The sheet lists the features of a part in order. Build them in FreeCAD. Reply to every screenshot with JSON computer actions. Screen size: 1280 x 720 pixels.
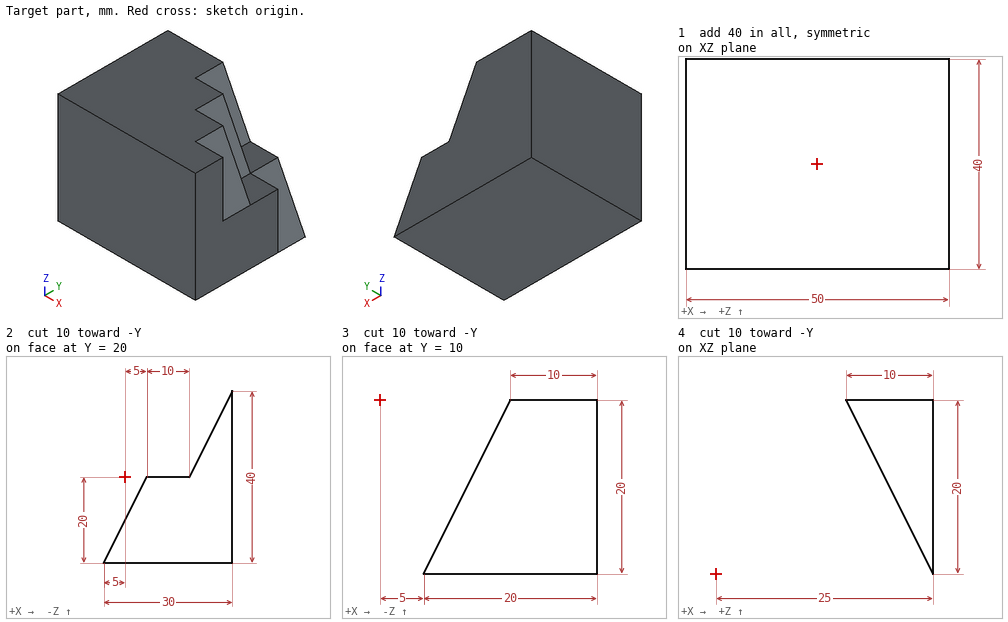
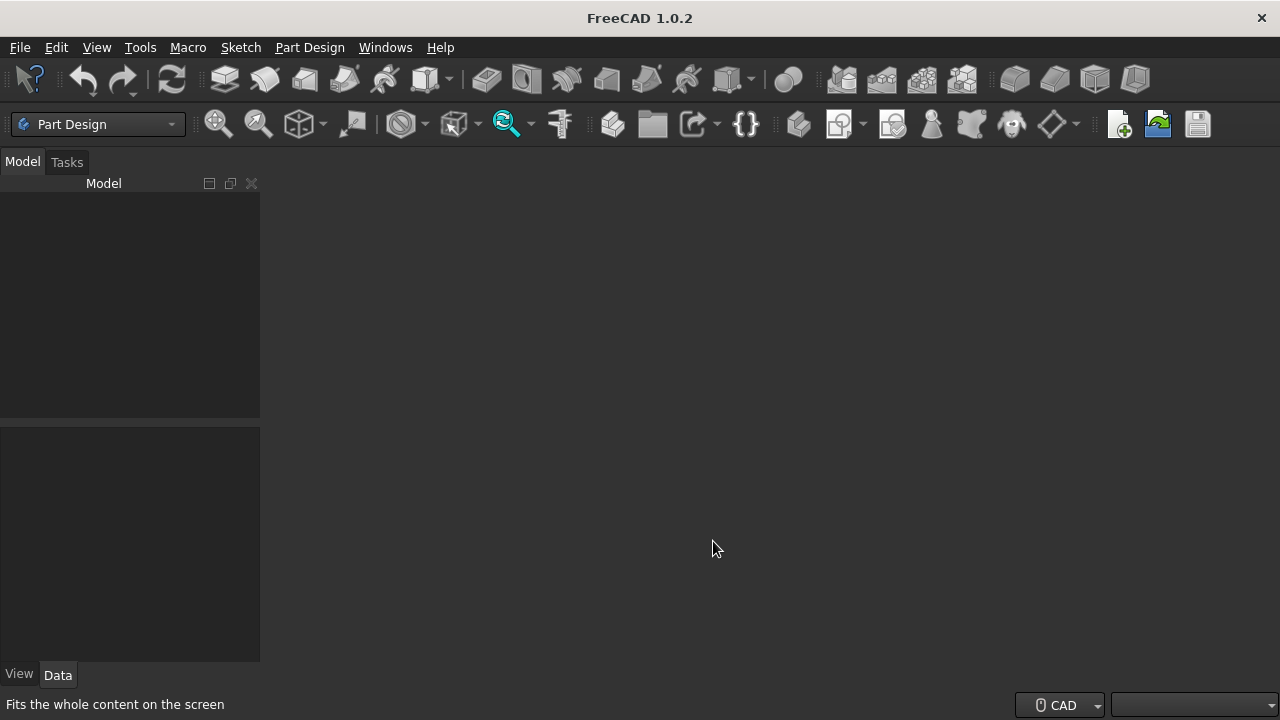
{"action": "left_click", "coordinate": [1118, 124]}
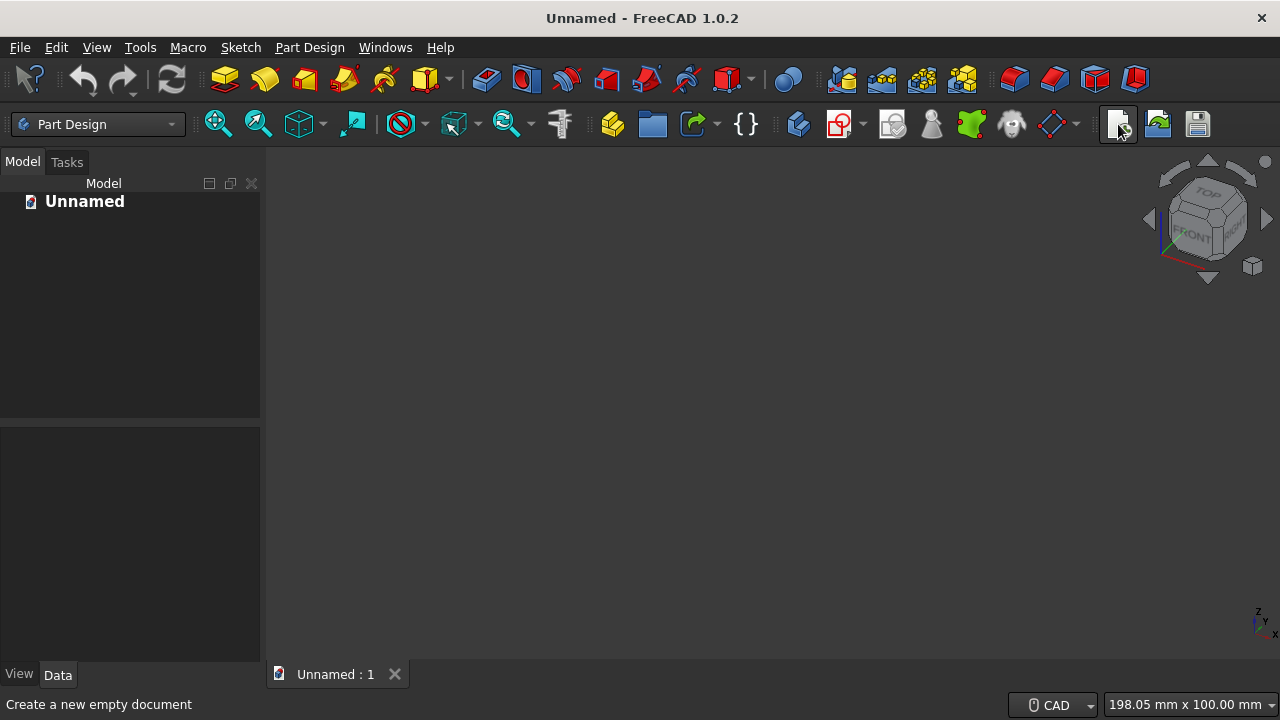
{"action": "left_click", "coordinate": [840, 124]}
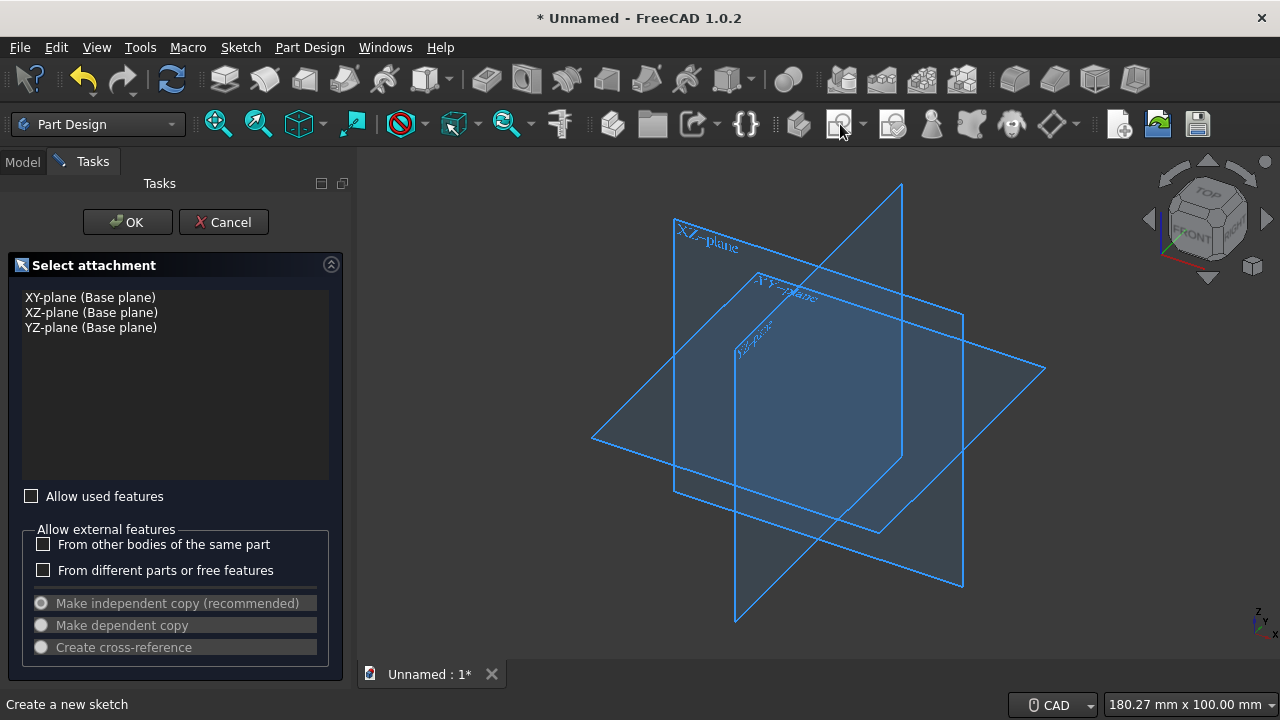
{"action": "left_click", "coordinate": [82, 312]}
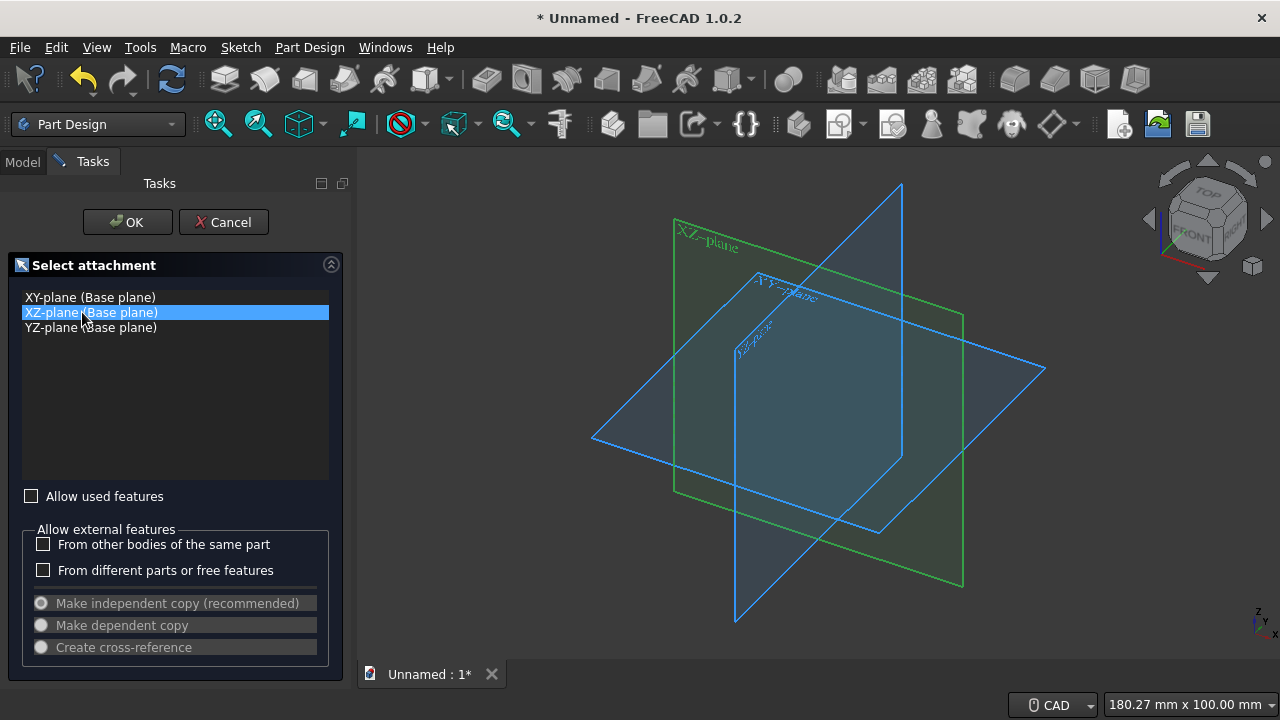
{"action": "left_click", "coordinate": [128, 222]}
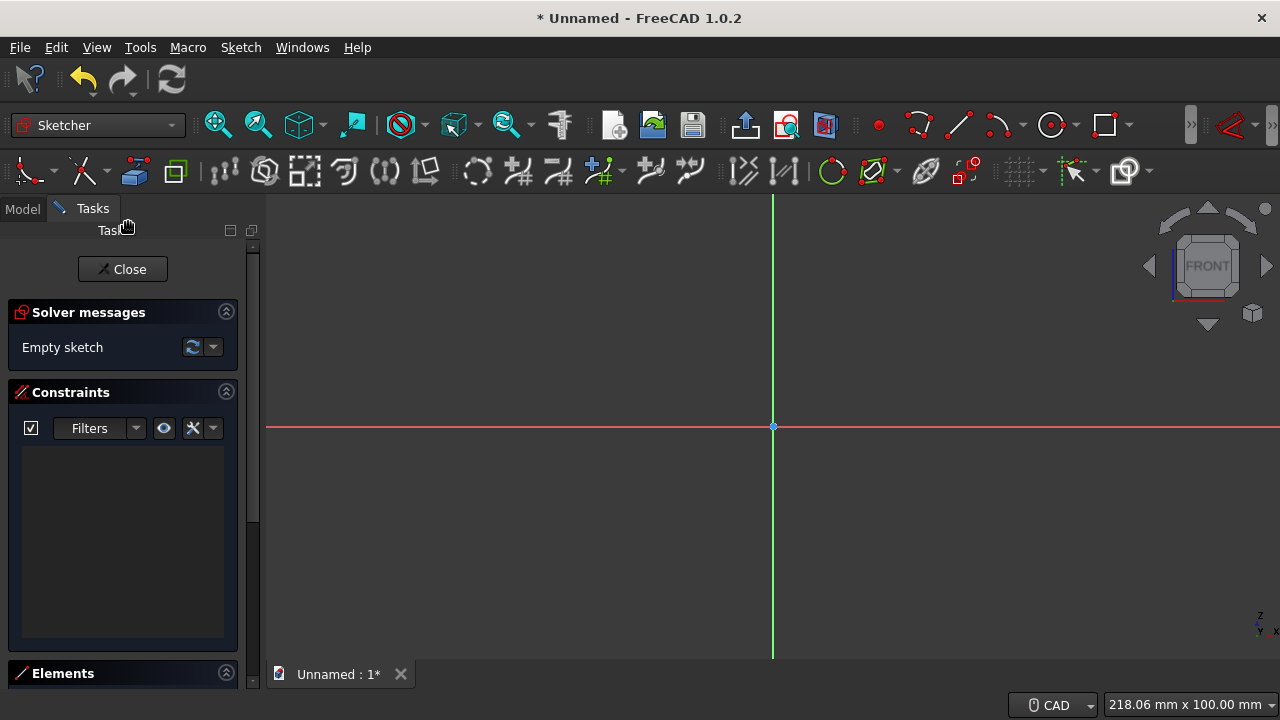
{"action": "scroll", "coordinate": [912, 426], "scroll_direction": "up", "scroll_amount": 2}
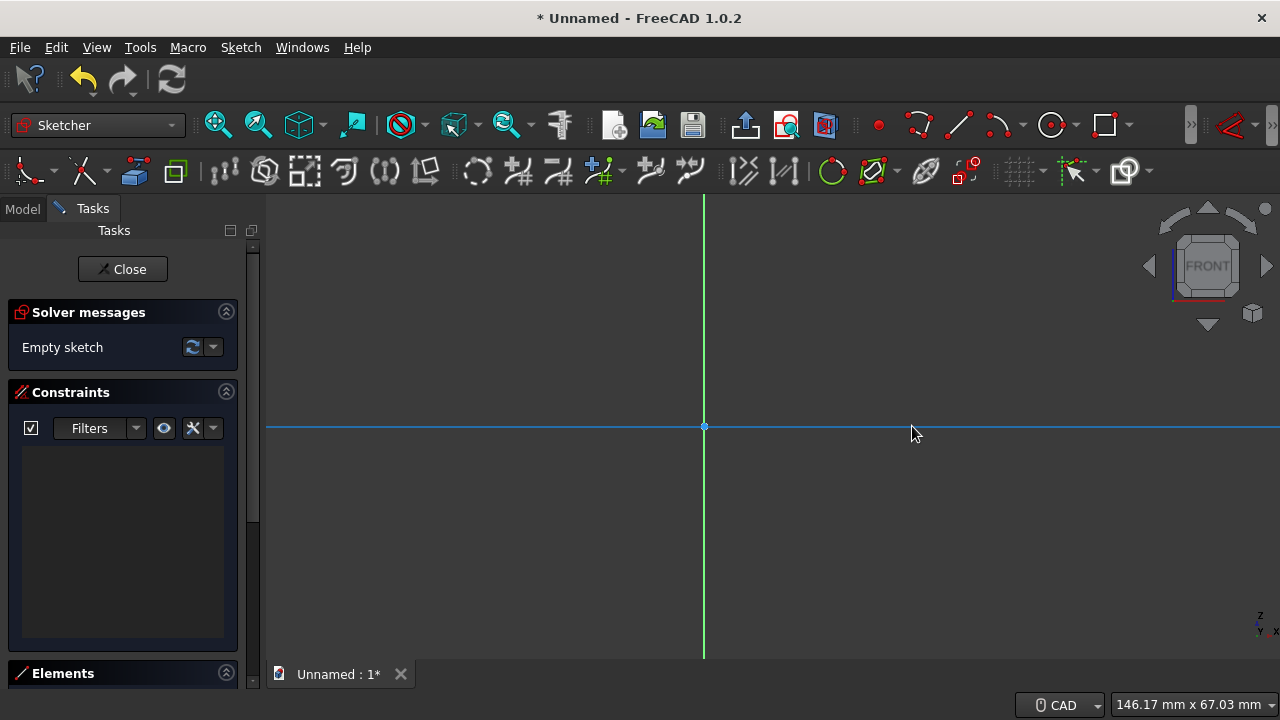
{"action": "left_click", "coordinate": [1132, 126]}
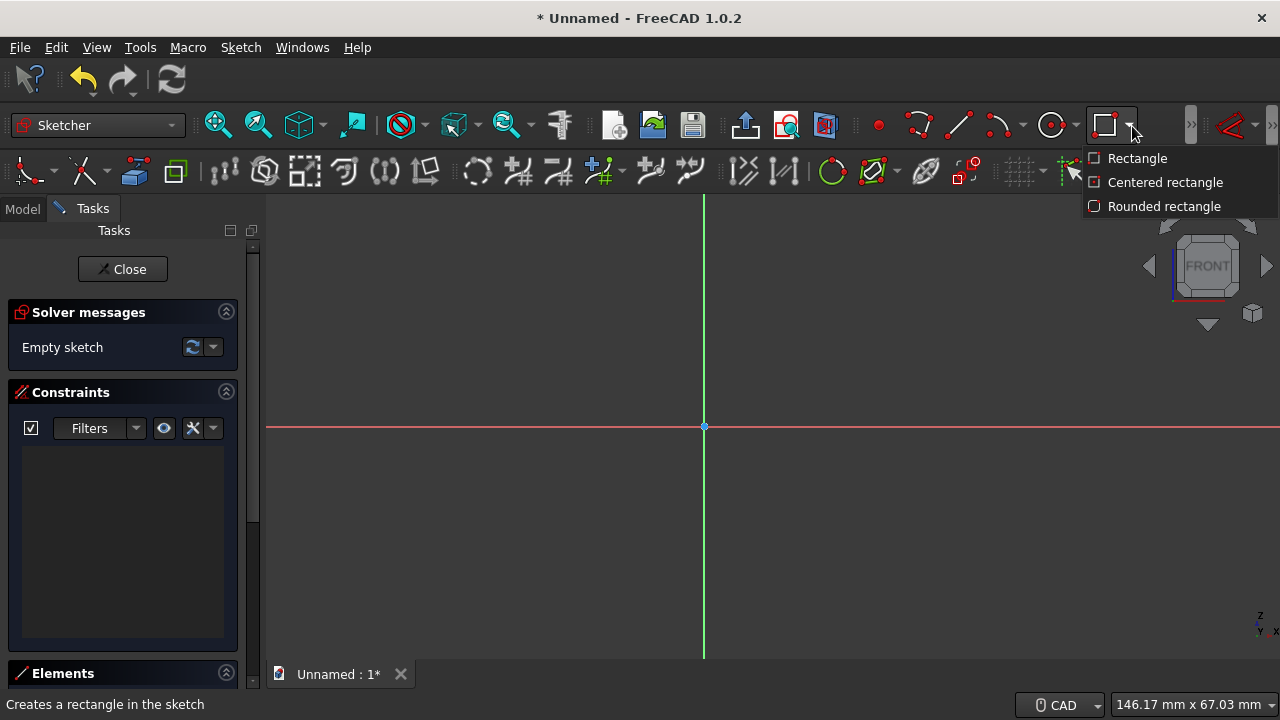
{"action": "left_click", "coordinate": [1180, 182]}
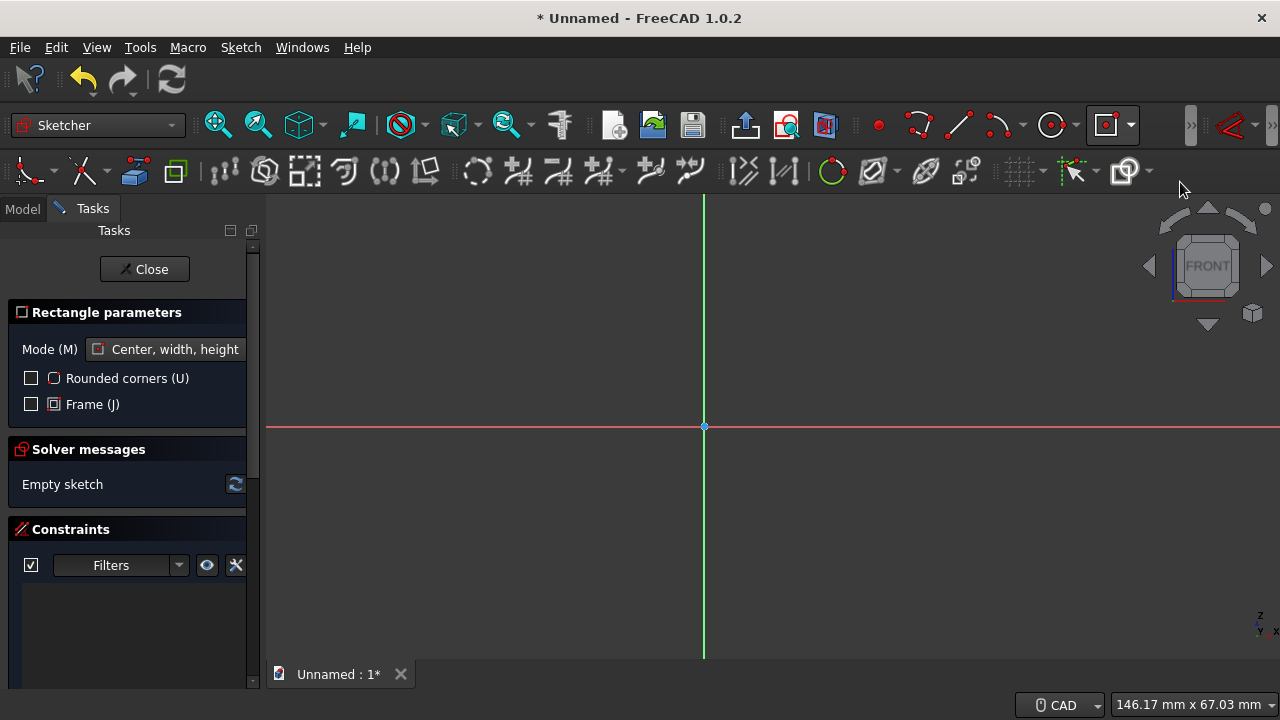
{"action": "left_click", "coordinate": [704, 426]}
{"action": "left_click", "coordinate": [878, 288]}
{"action": "key", "text": "Escape"}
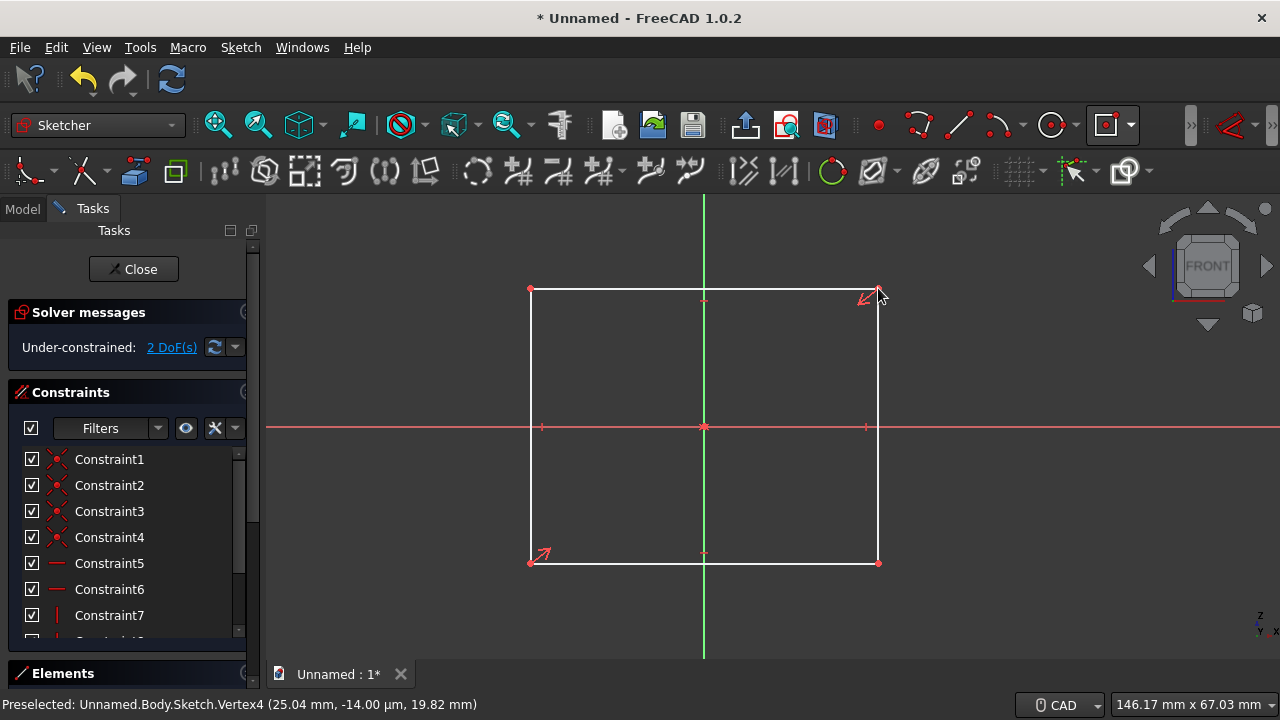
{"action": "left_click", "coordinate": [1230, 126]}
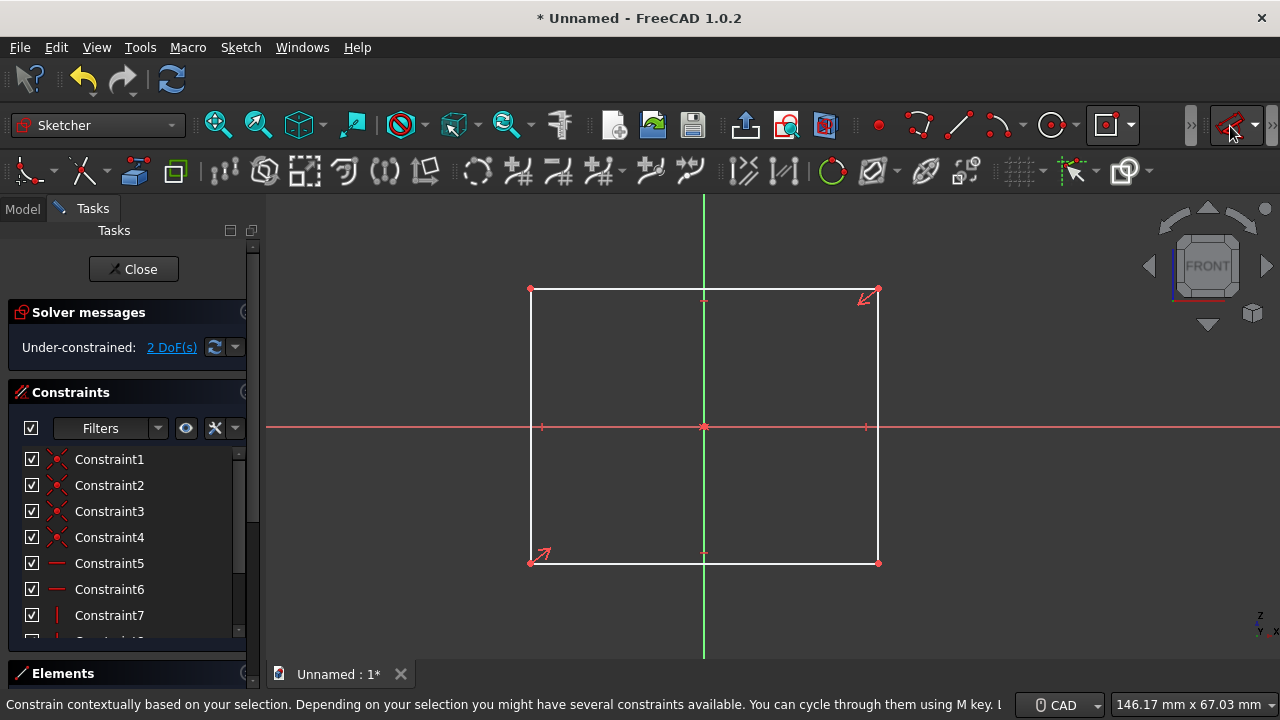
{"action": "left_click", "coordinate": [635, 564]}
{"action": "left_click", "coordinate": [624, 598]}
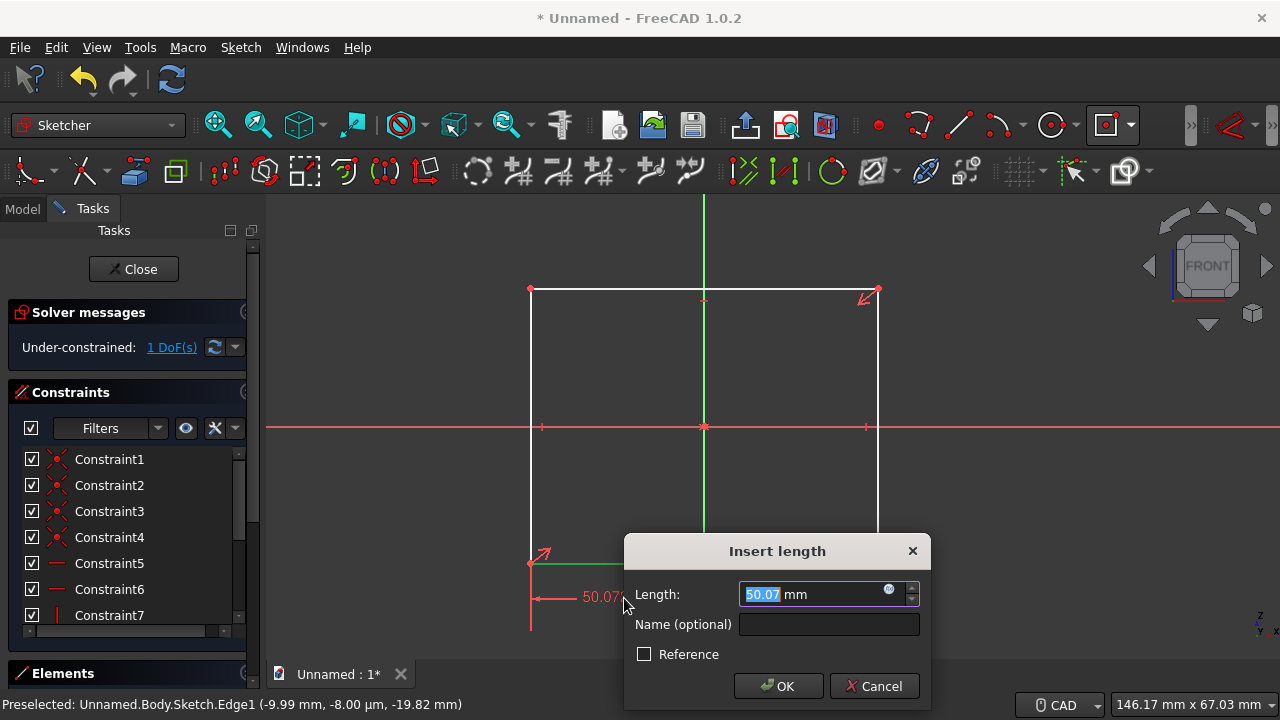
{"action": "type", "text": "50"}
{"action": "key", "text": "Return"}